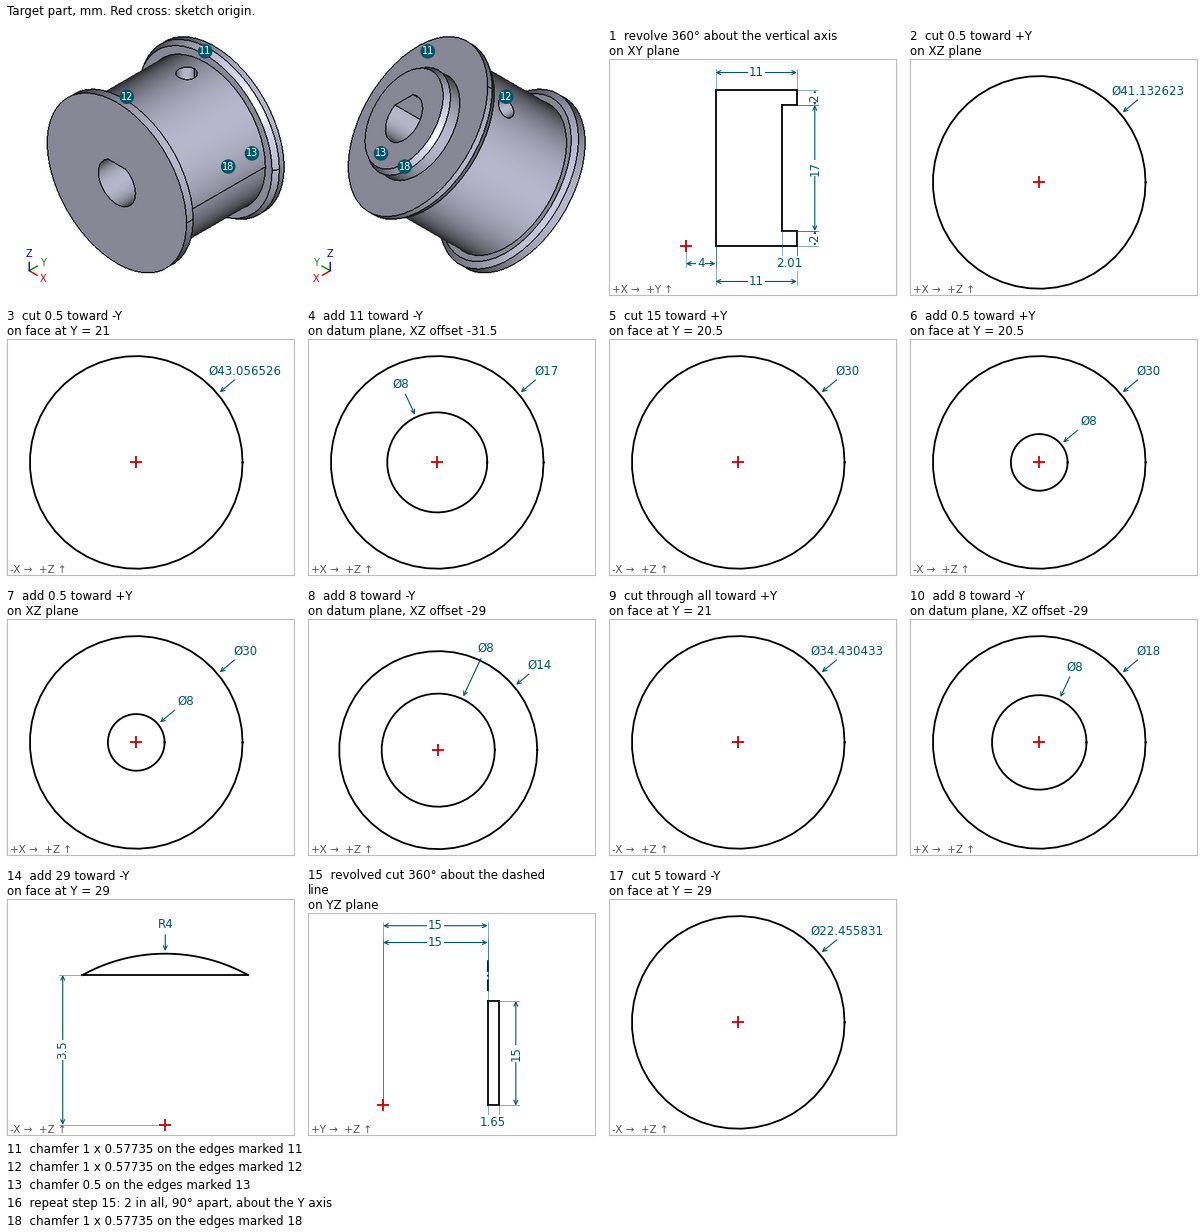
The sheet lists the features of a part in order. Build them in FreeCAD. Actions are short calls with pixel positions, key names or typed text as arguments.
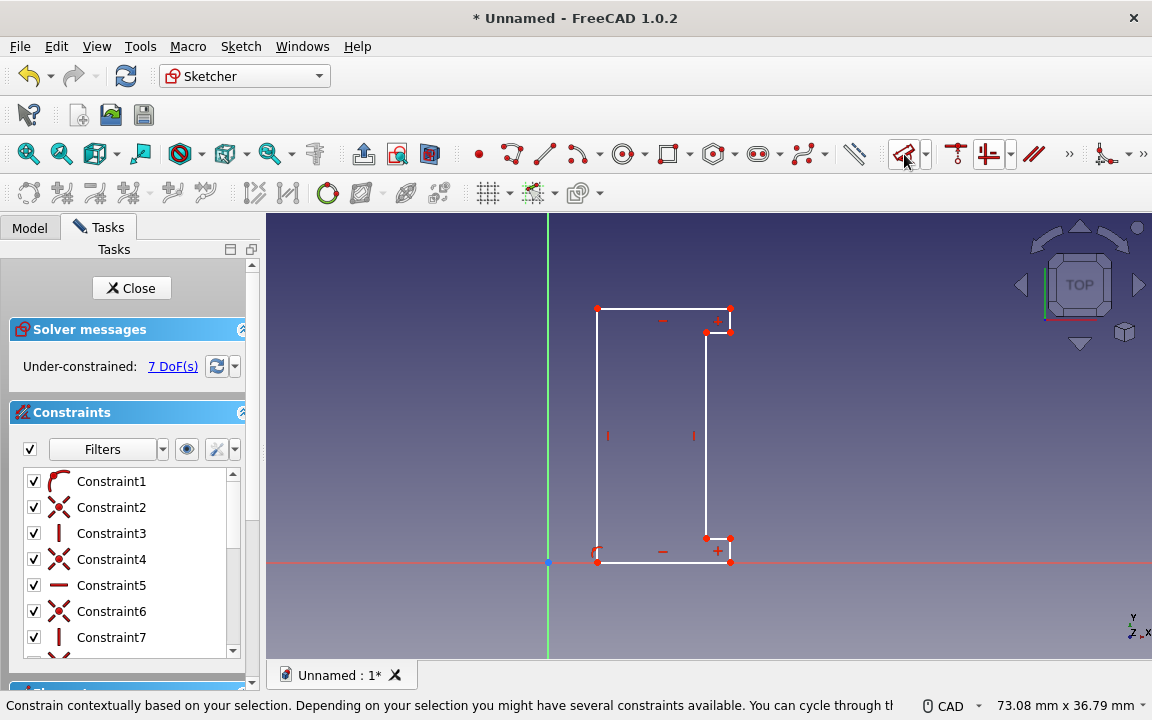
scroll(730, 553, up, 3)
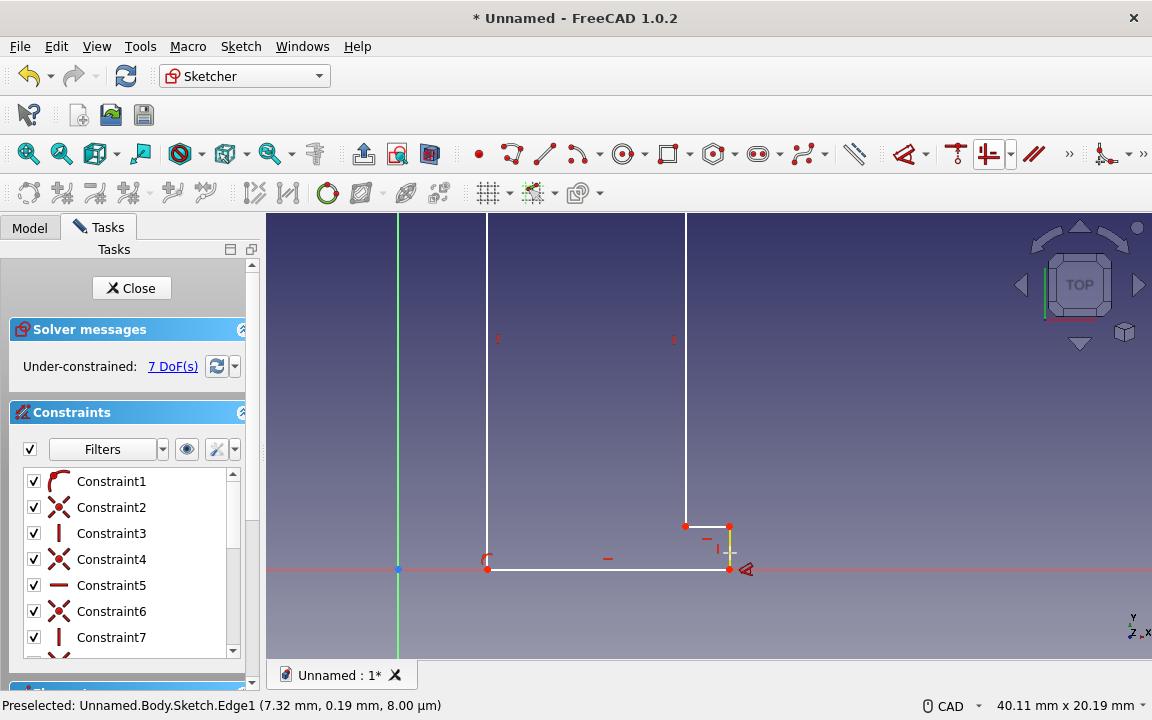
click(730, 553)
click(764, 548)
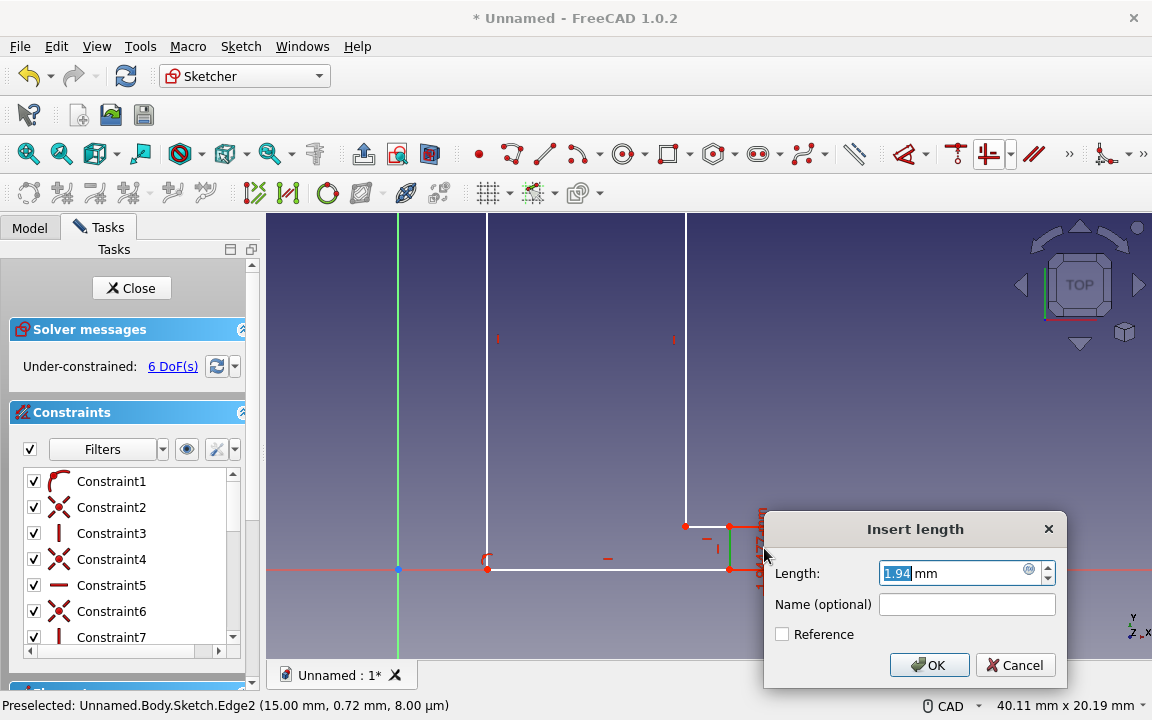
text(2)
key(Return)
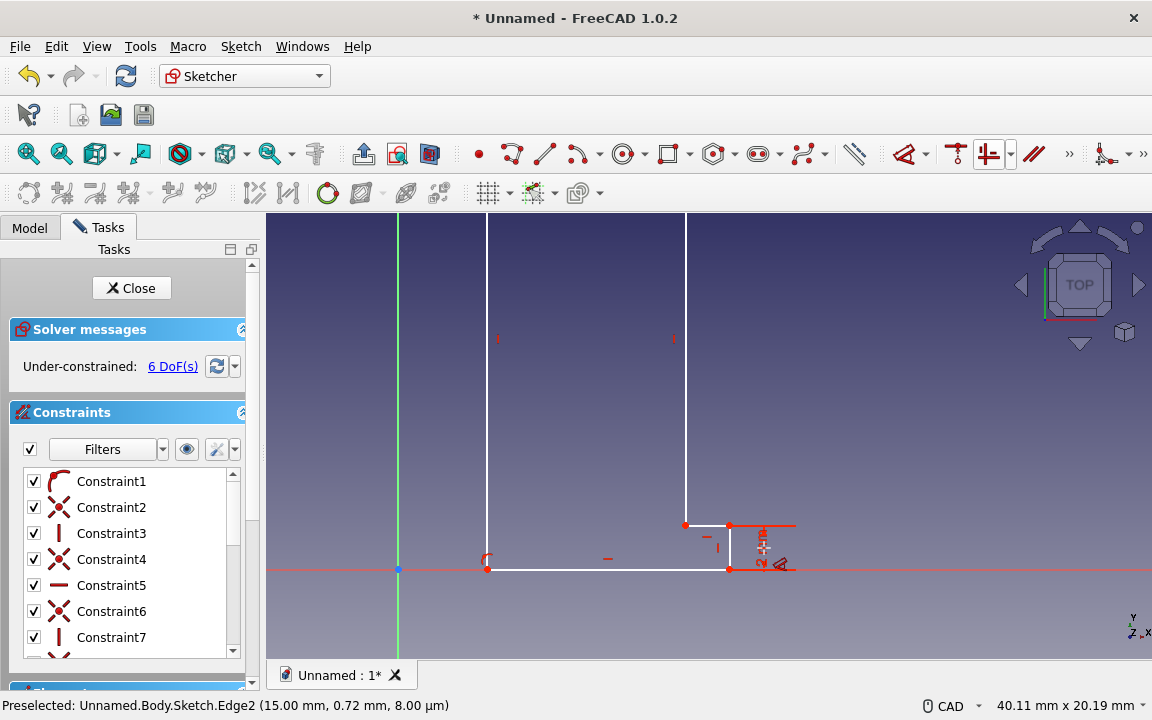
scroll(734, 555, down, 3)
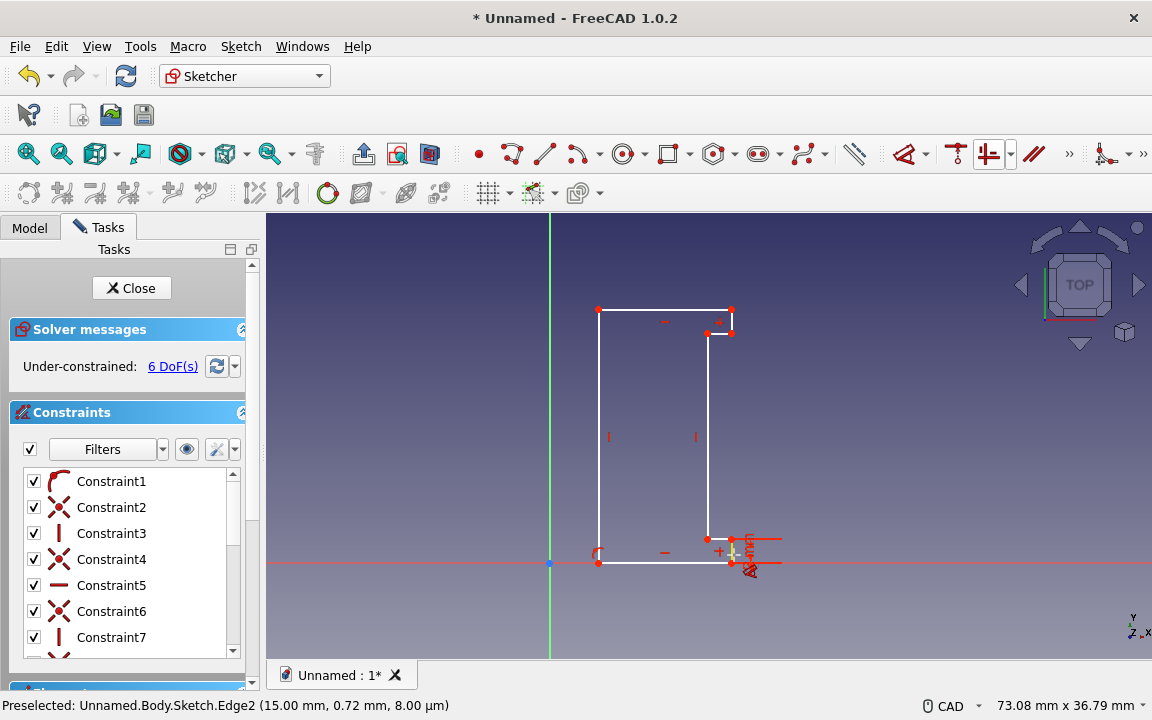
scroll(732, 327, up, 4)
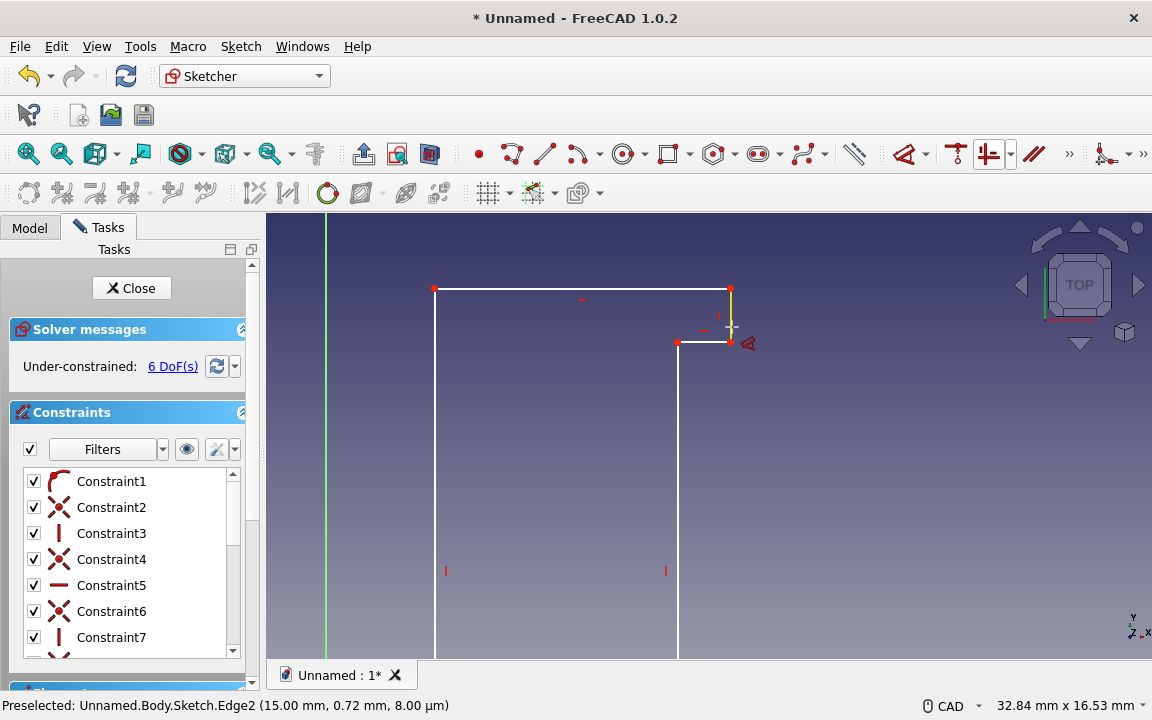
click(731, 326)
click(765, 315)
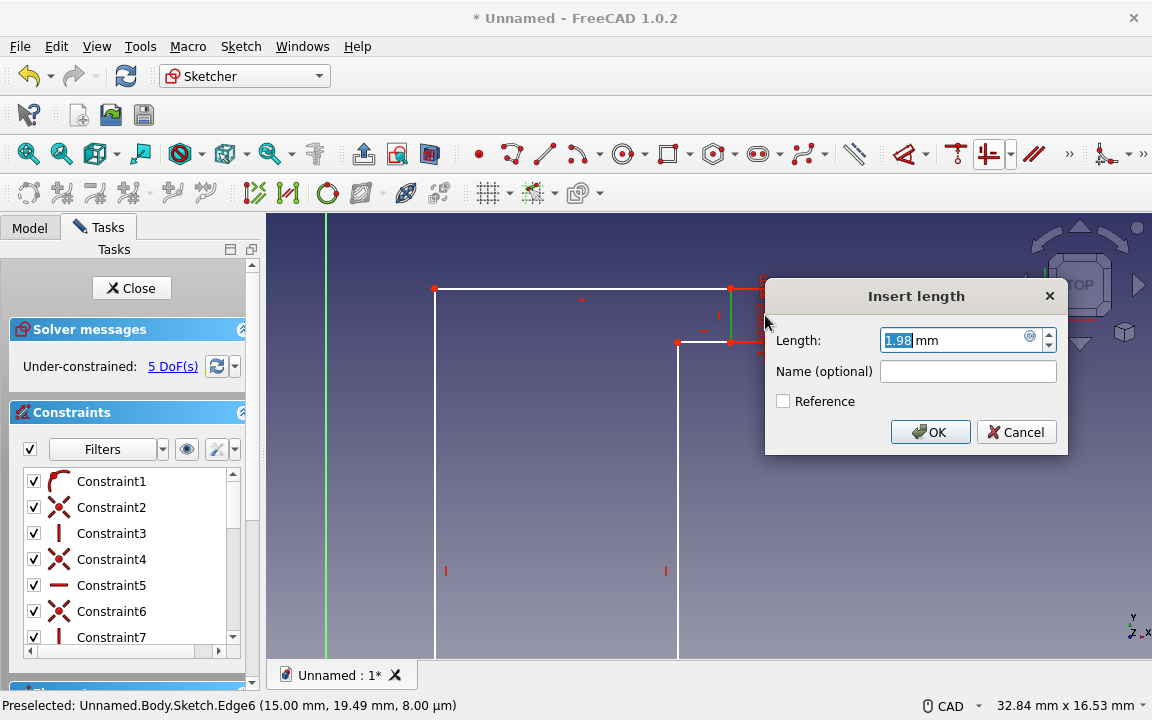
text(2)
key(Return)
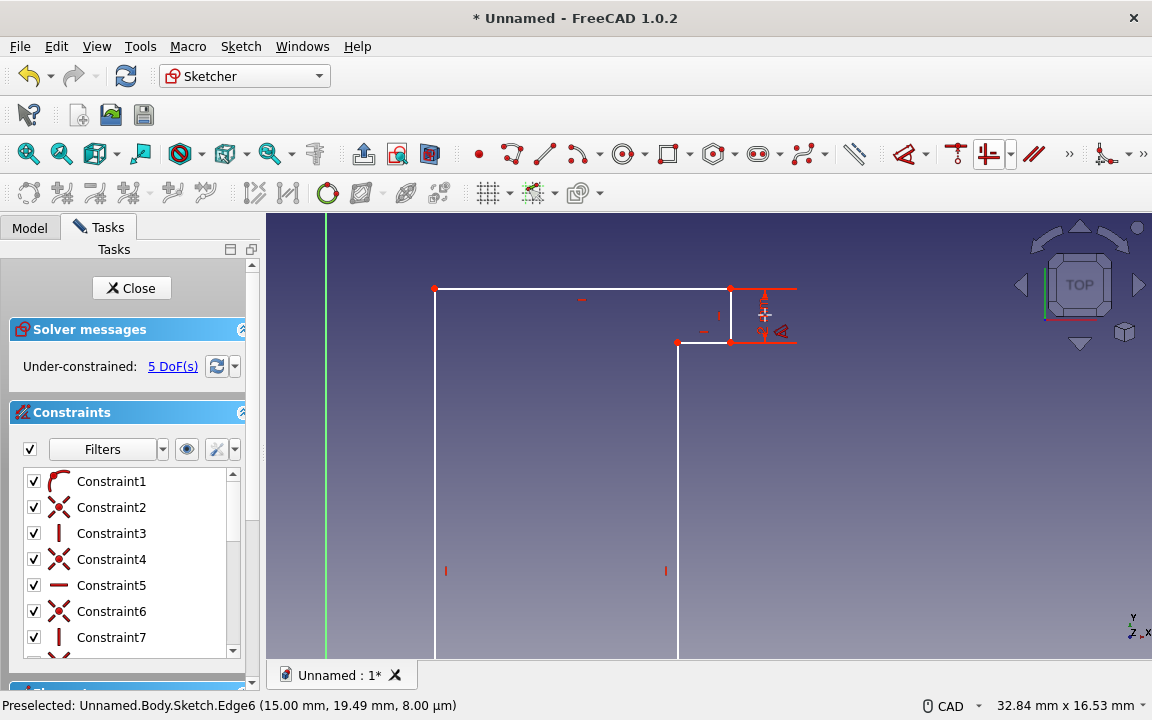
scroll(732, 327, down, 4)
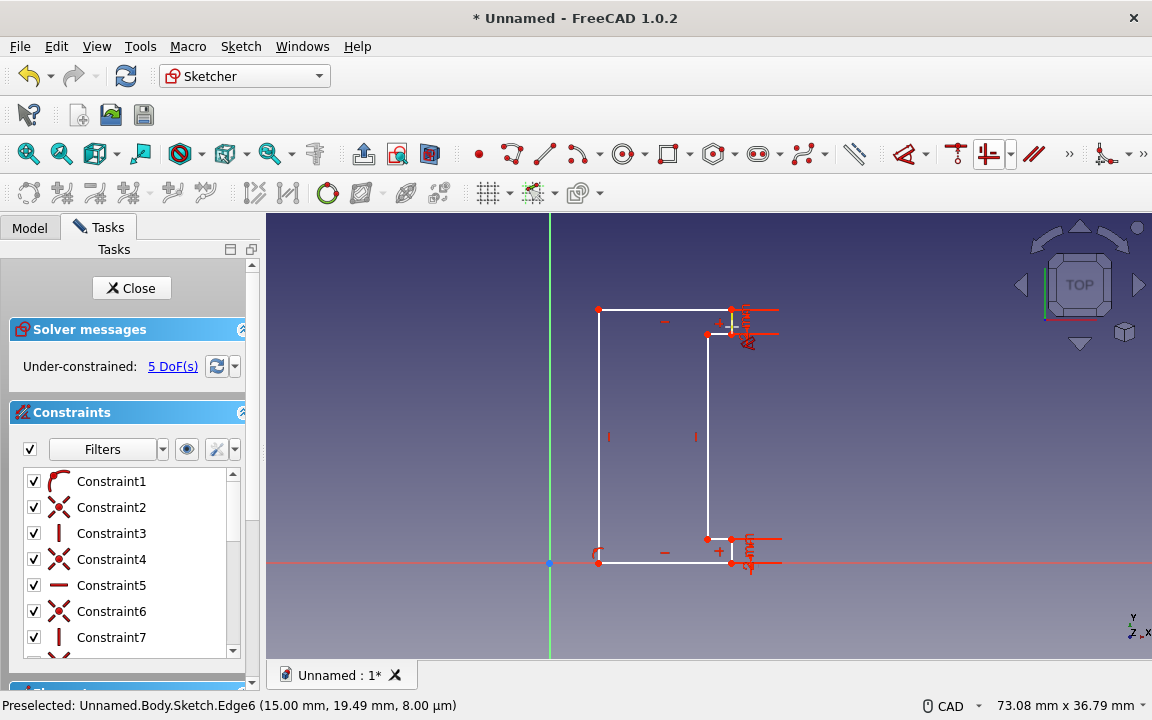
click(639, 563)
click(665, 597)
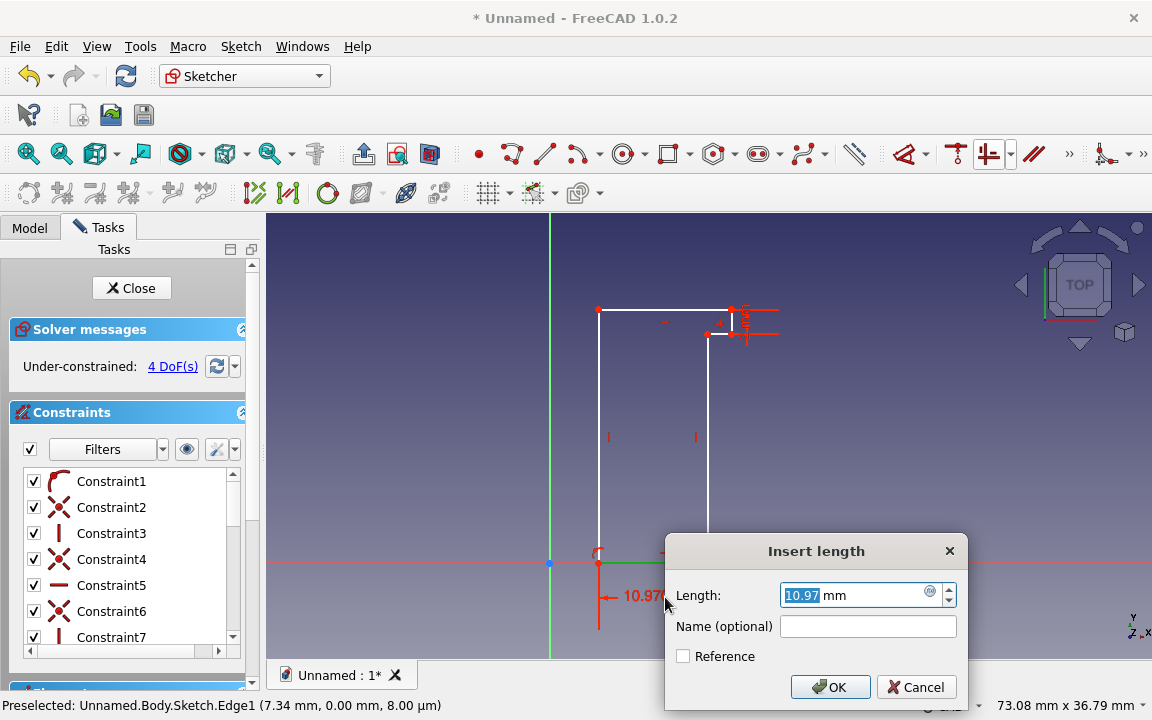
text(11)
key(Return)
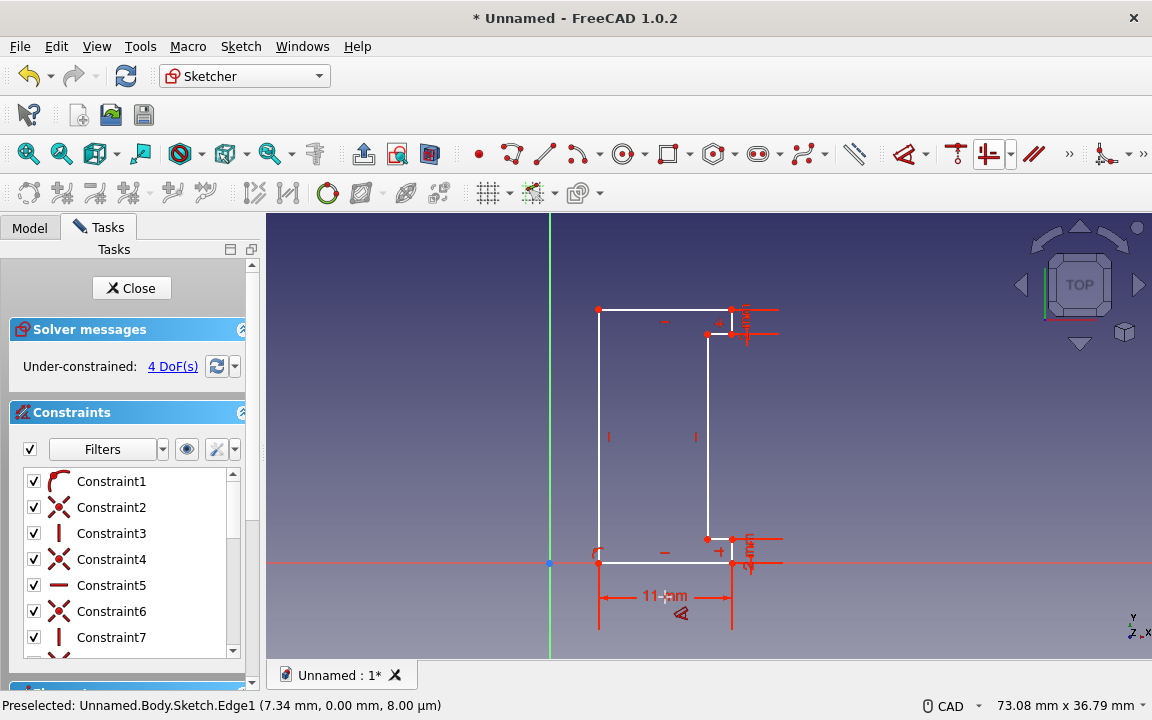
click(708, 478)
click(742, 437)